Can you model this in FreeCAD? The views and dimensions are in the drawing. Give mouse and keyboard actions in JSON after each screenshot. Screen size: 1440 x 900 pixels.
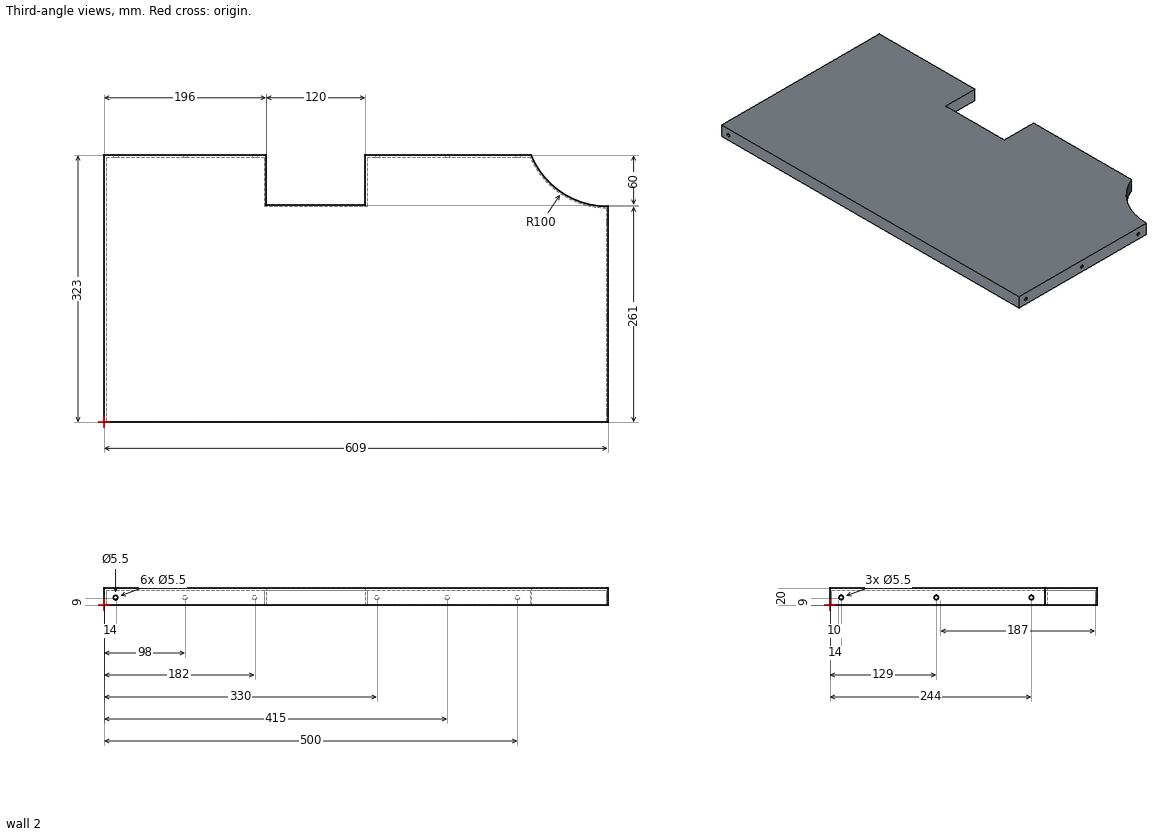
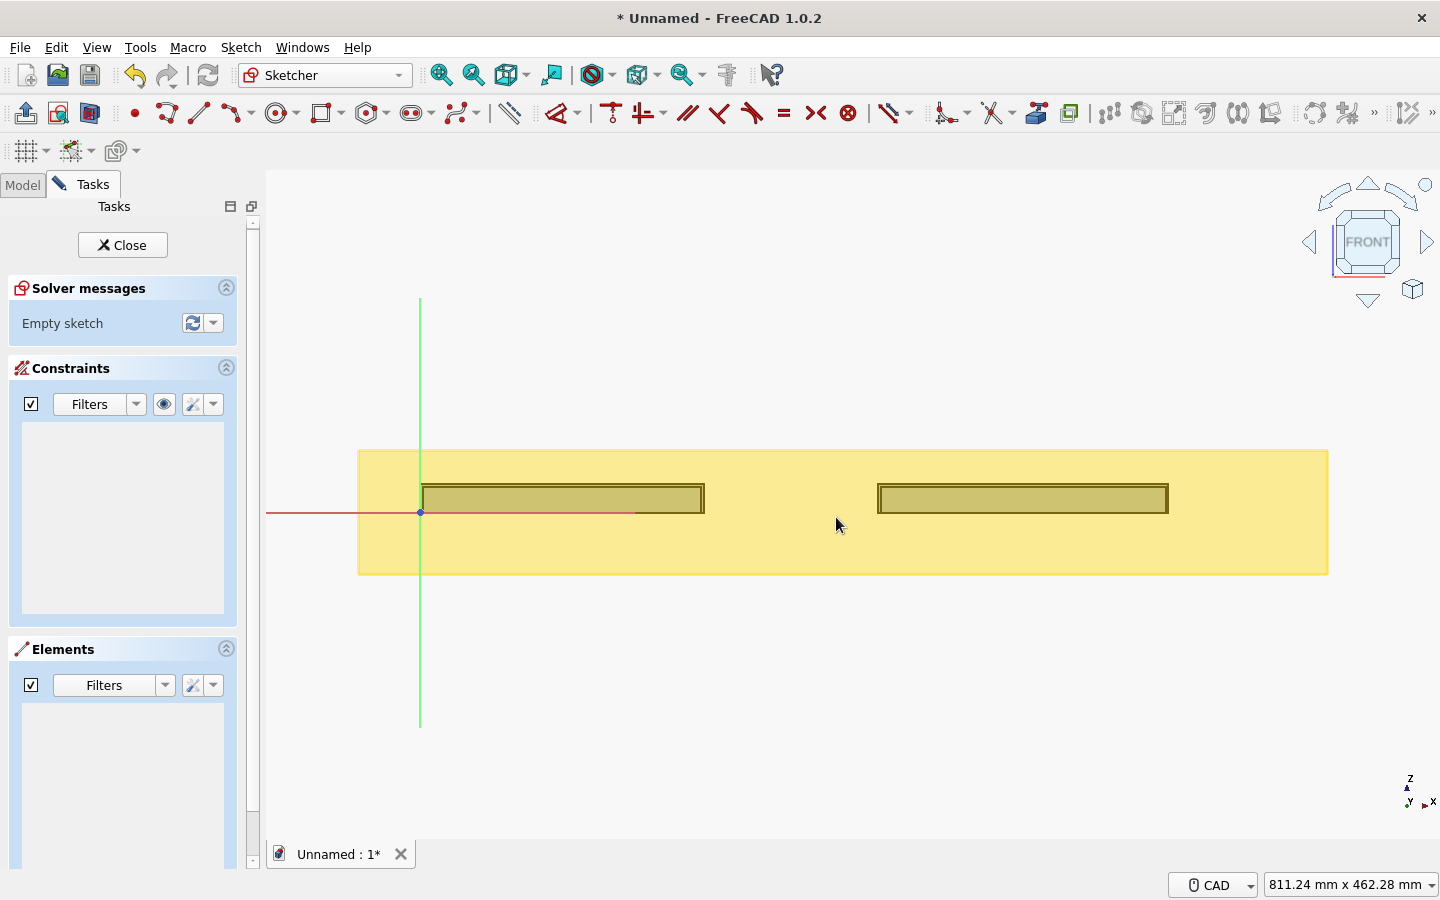
{"action": "left_click", "coordinate": [276, 114]}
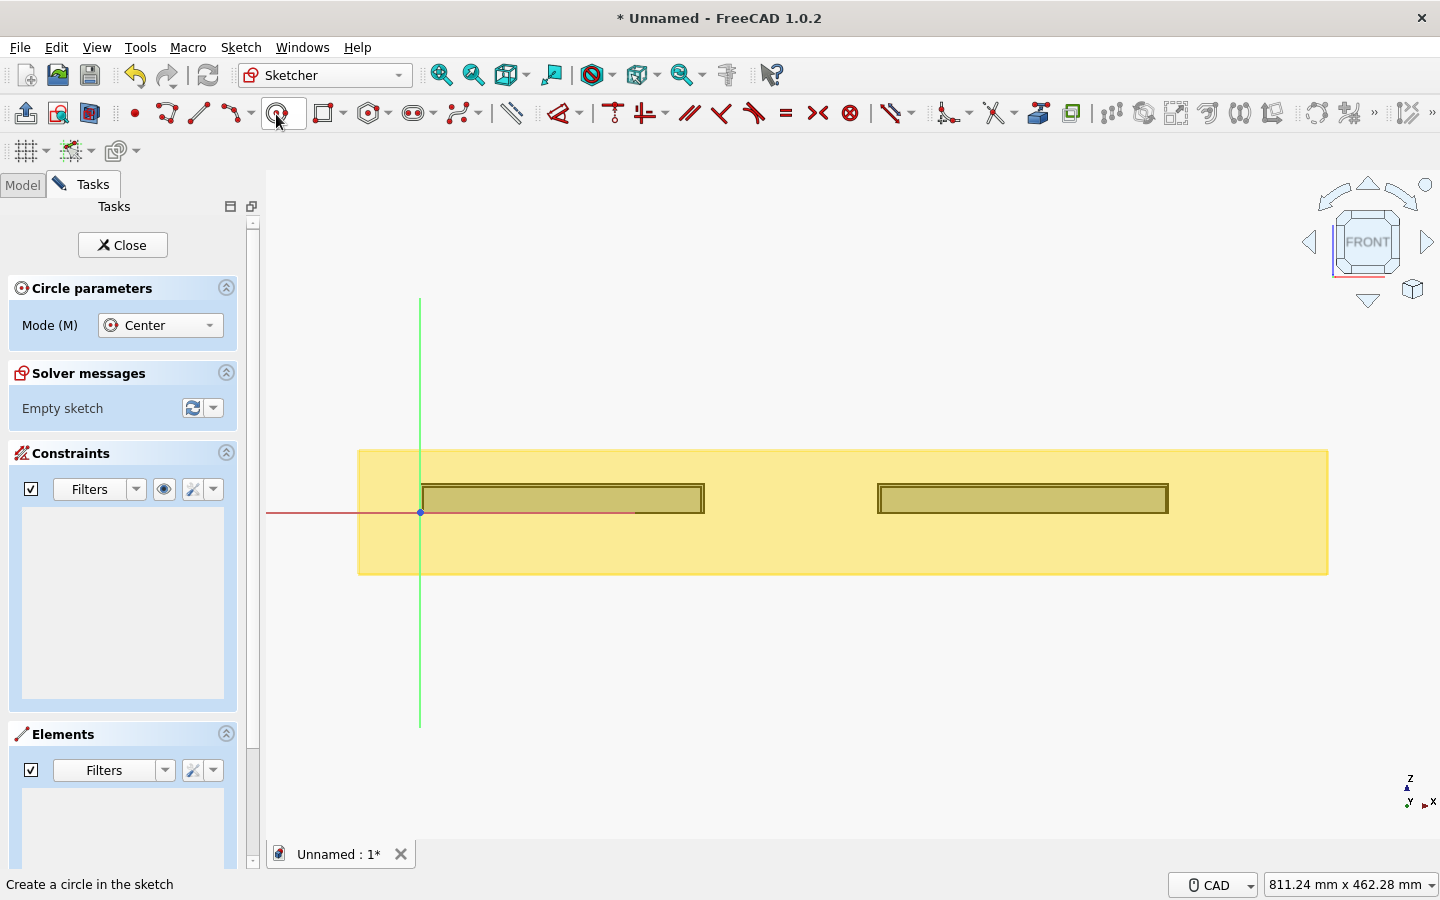
{"action": "scroll", "coordinate": [441, 500], "scroll_direction": "up", "scroll_amount": 9}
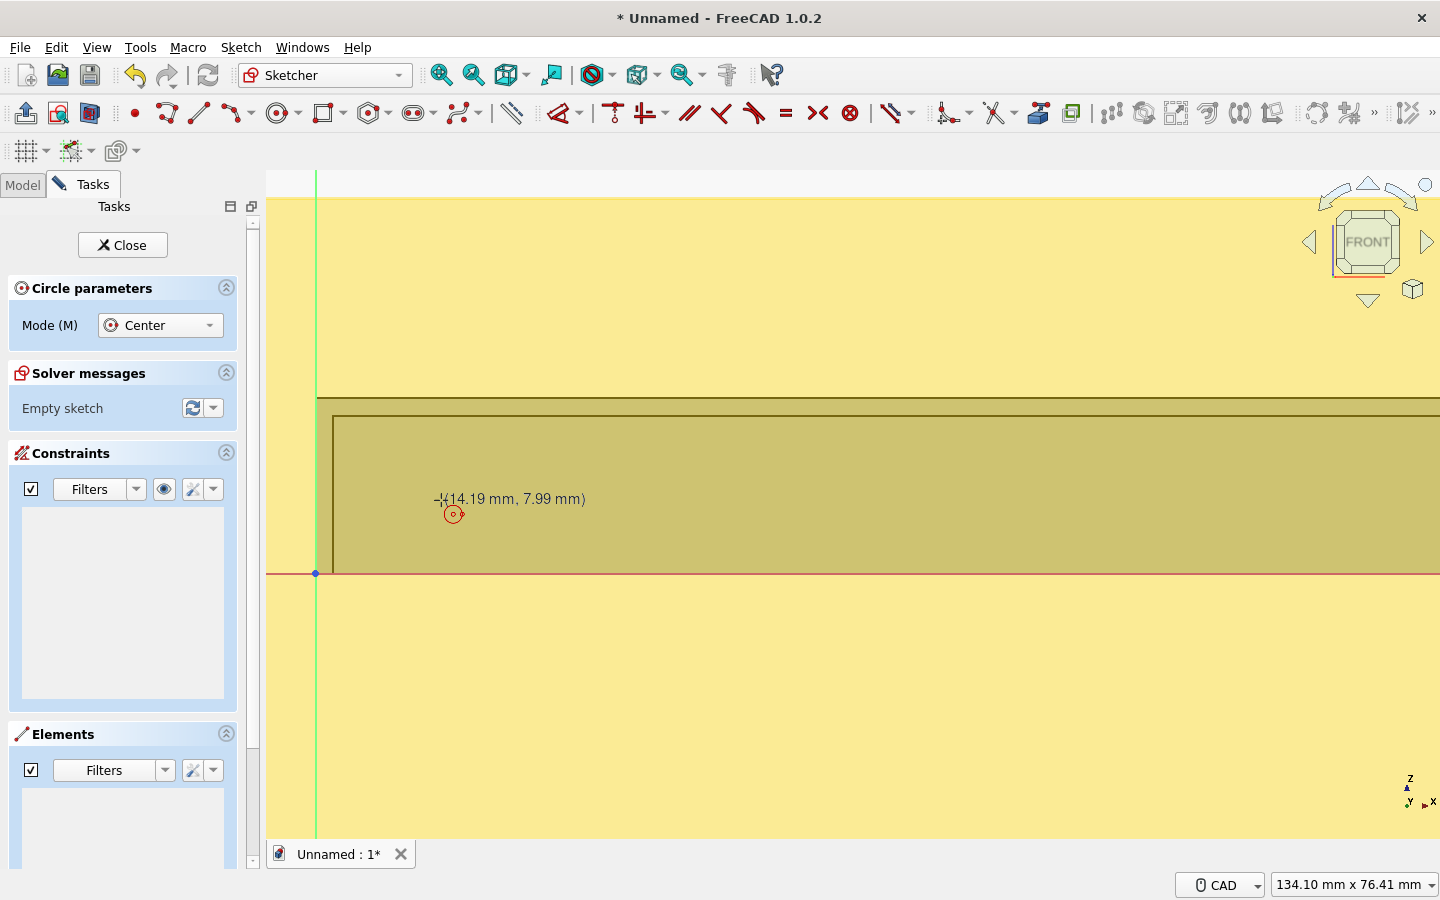
{"action": "scroll", "coordinate": [441, 501], "scroll_direction": "down", "scroll_amount": 9}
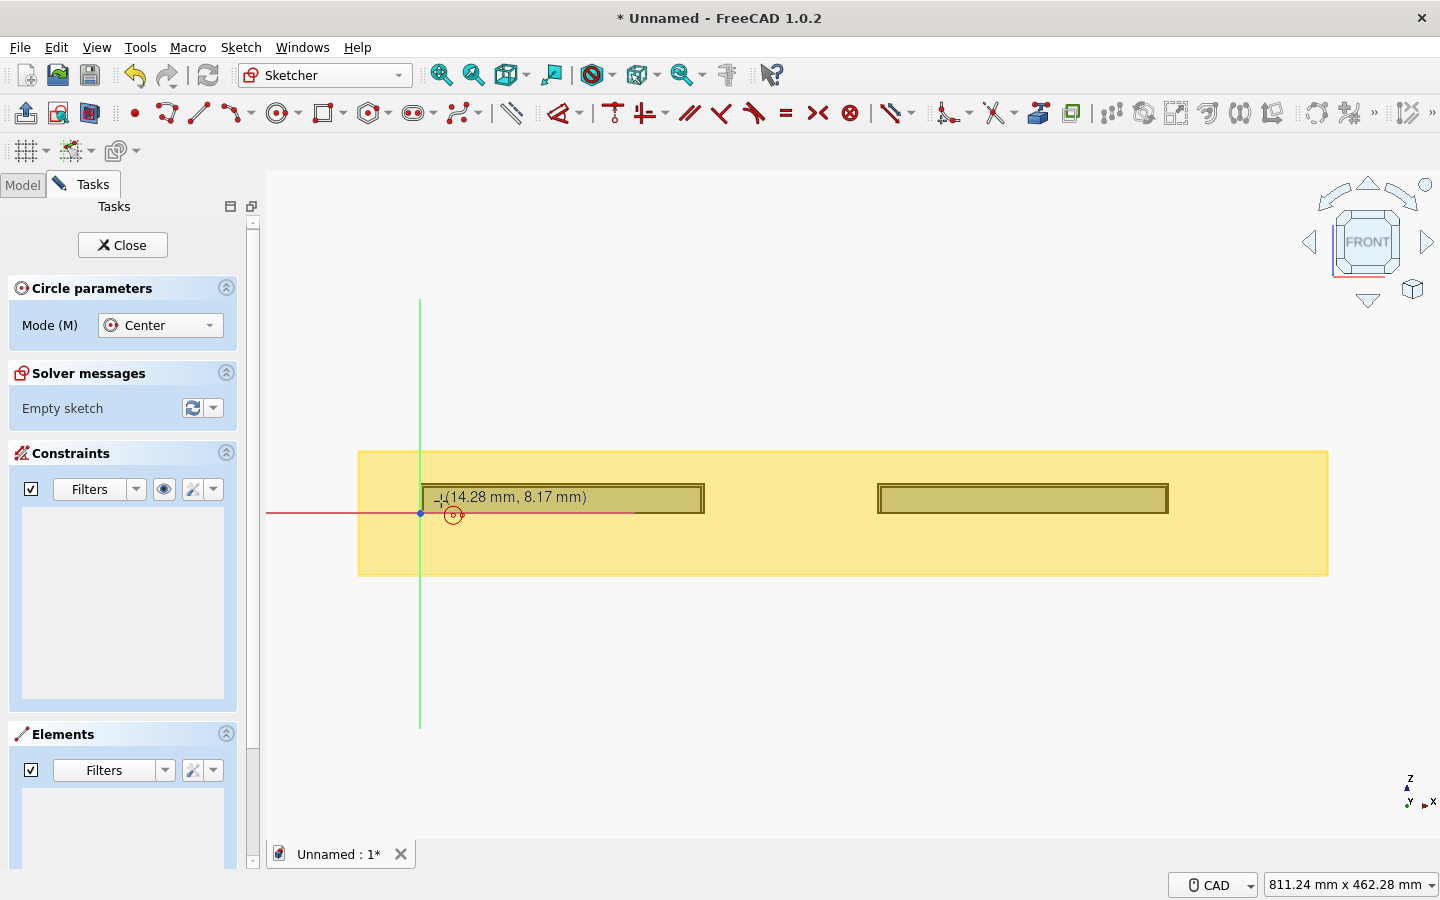
{"action": "left_click", "coordinate": [441, 500]}
{"action": "mouse_move", "coordinate": [444, 498]}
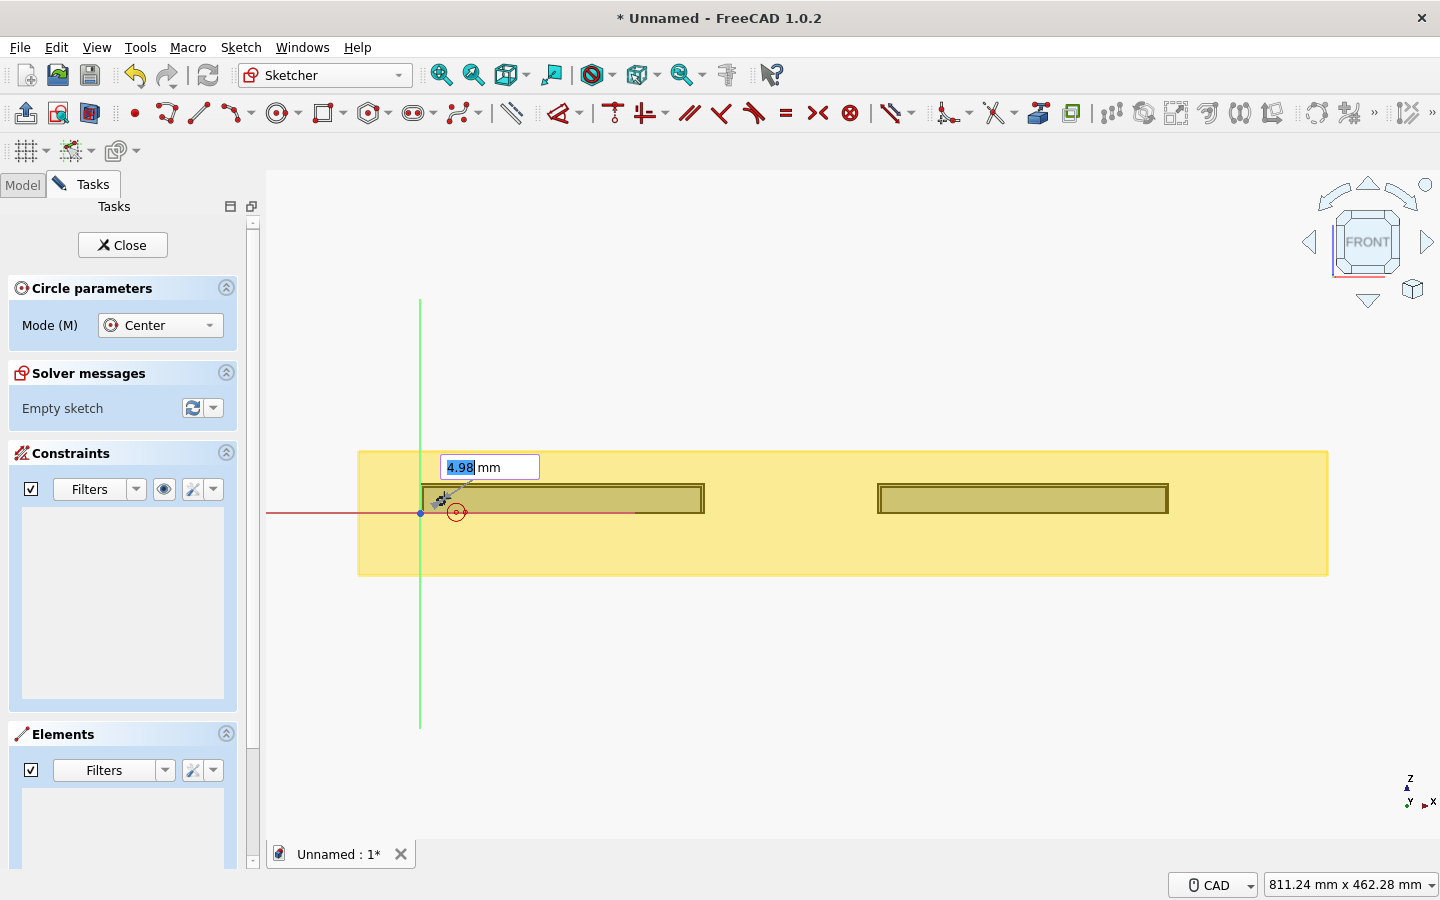
{"action": "type", "text": "5.5"}
{"action": "key", "text": "Return"}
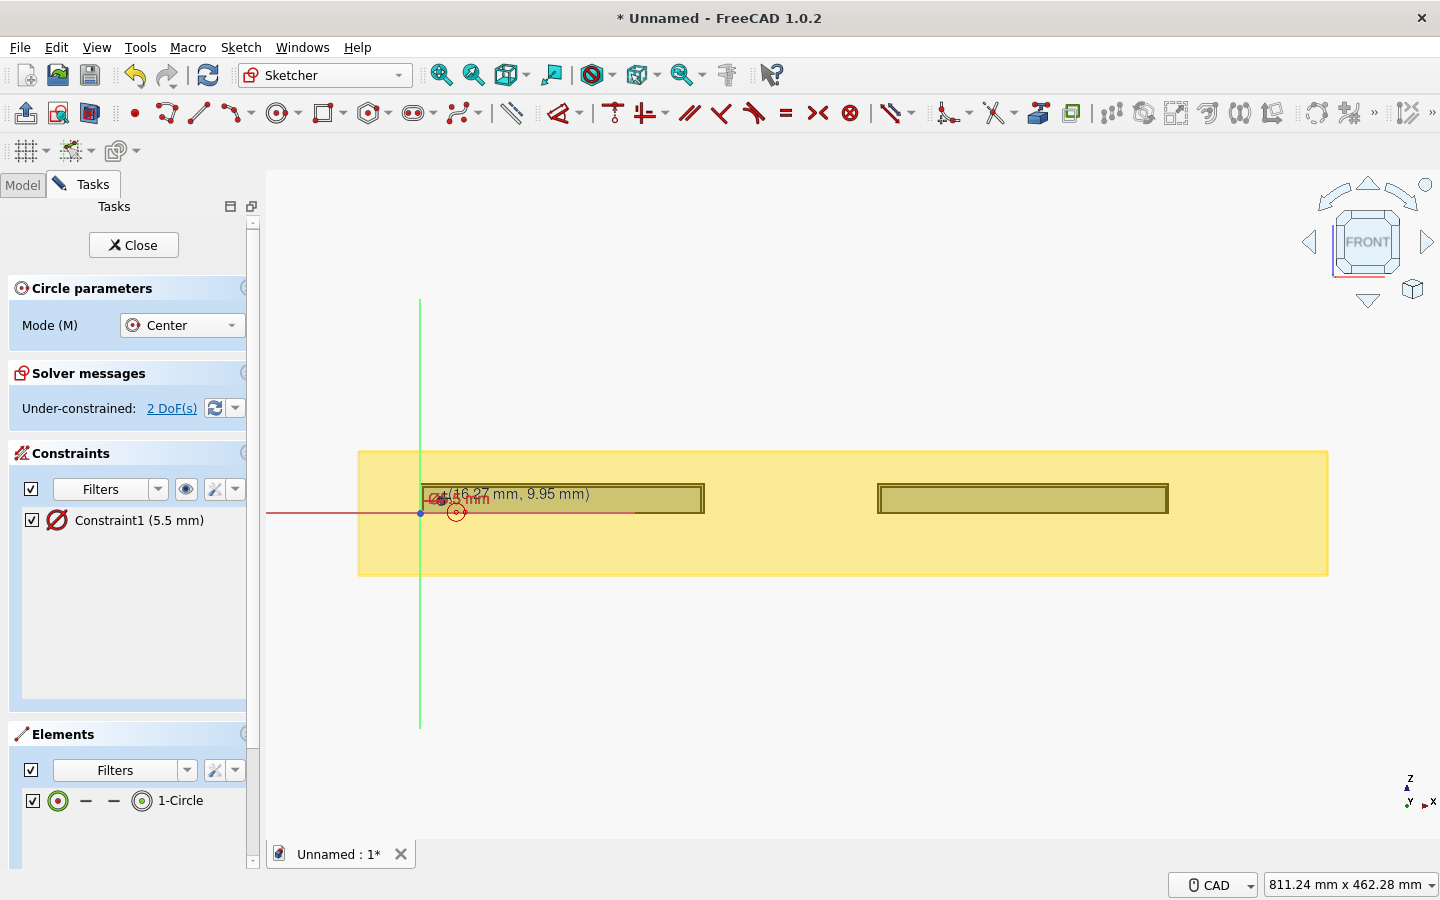
{"action": "scroll", "coordinate": [684, 500], "scroll_direction": "up", "scroll_amount": 9}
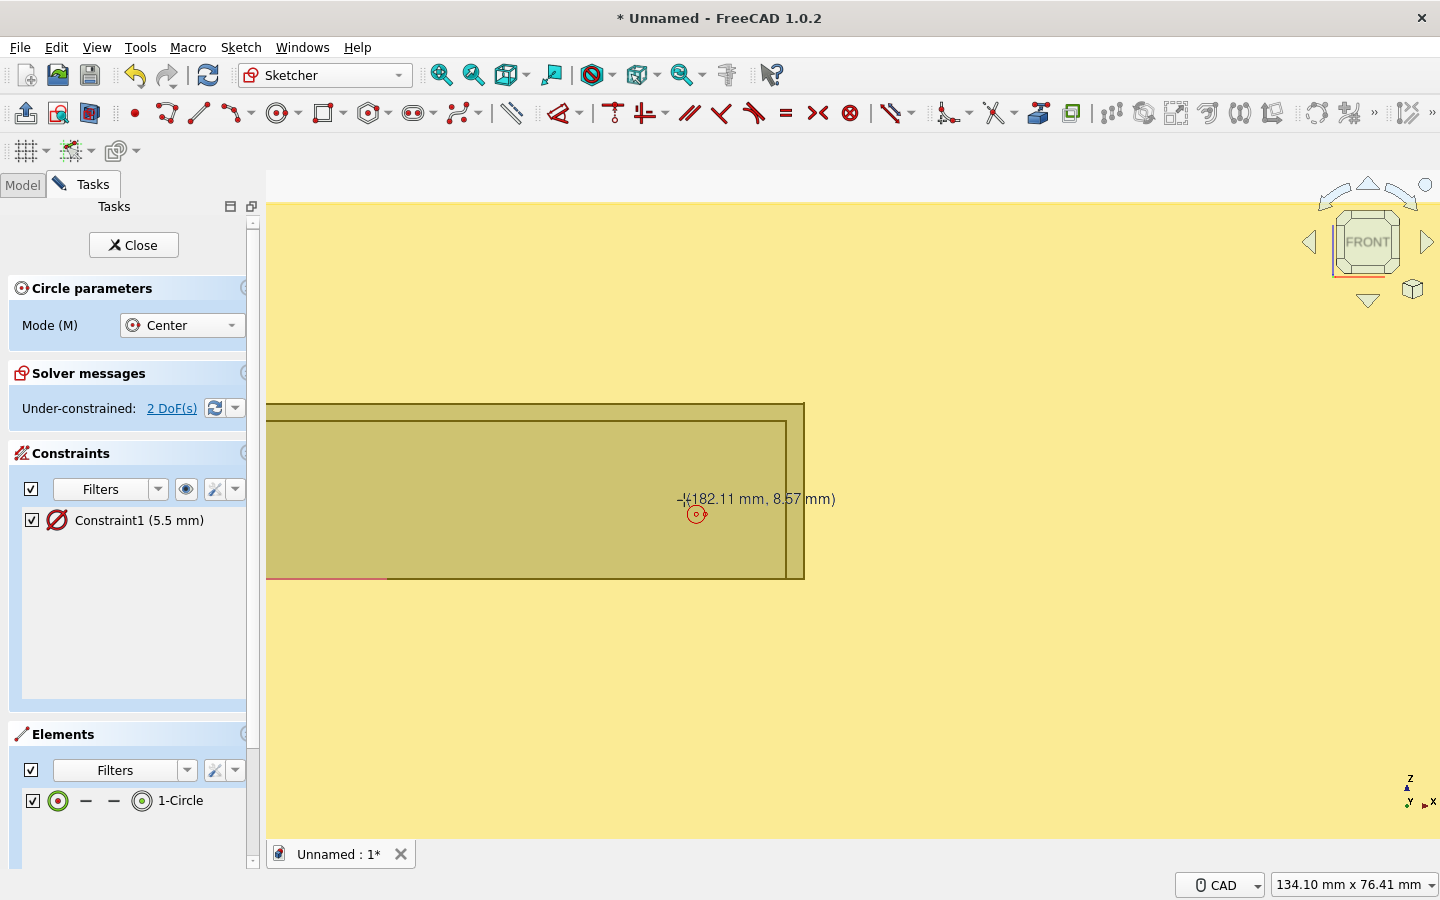
{"action": "scroll", "coordinate": [685, 500], "scroll_direction": "down", "scroll_amount": 9}